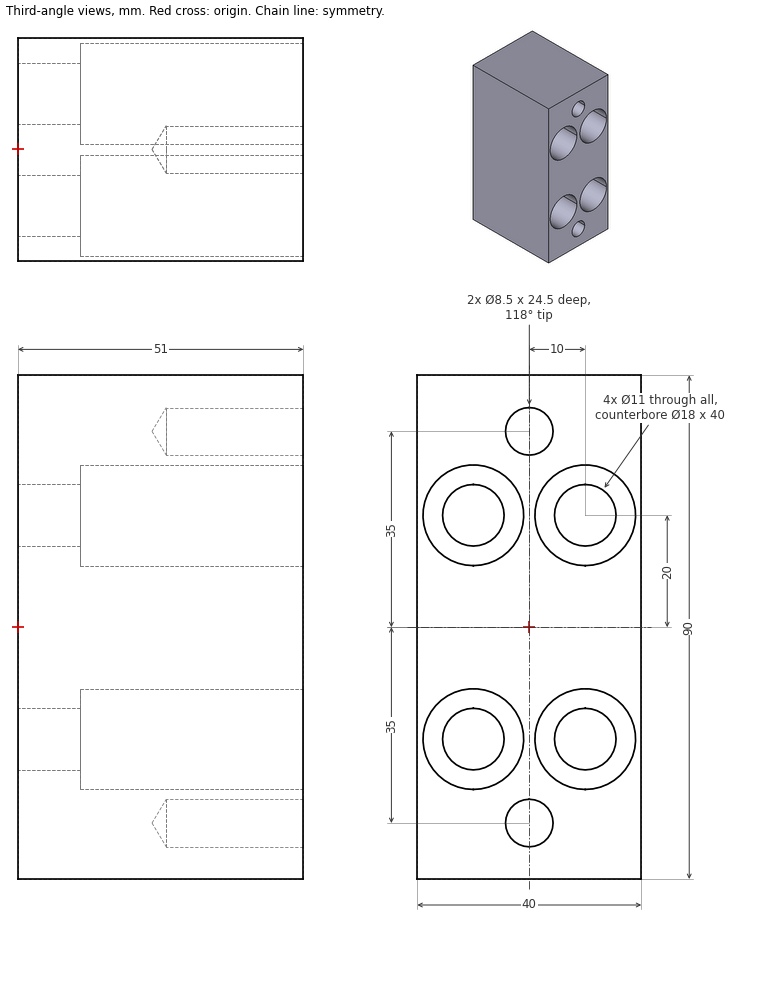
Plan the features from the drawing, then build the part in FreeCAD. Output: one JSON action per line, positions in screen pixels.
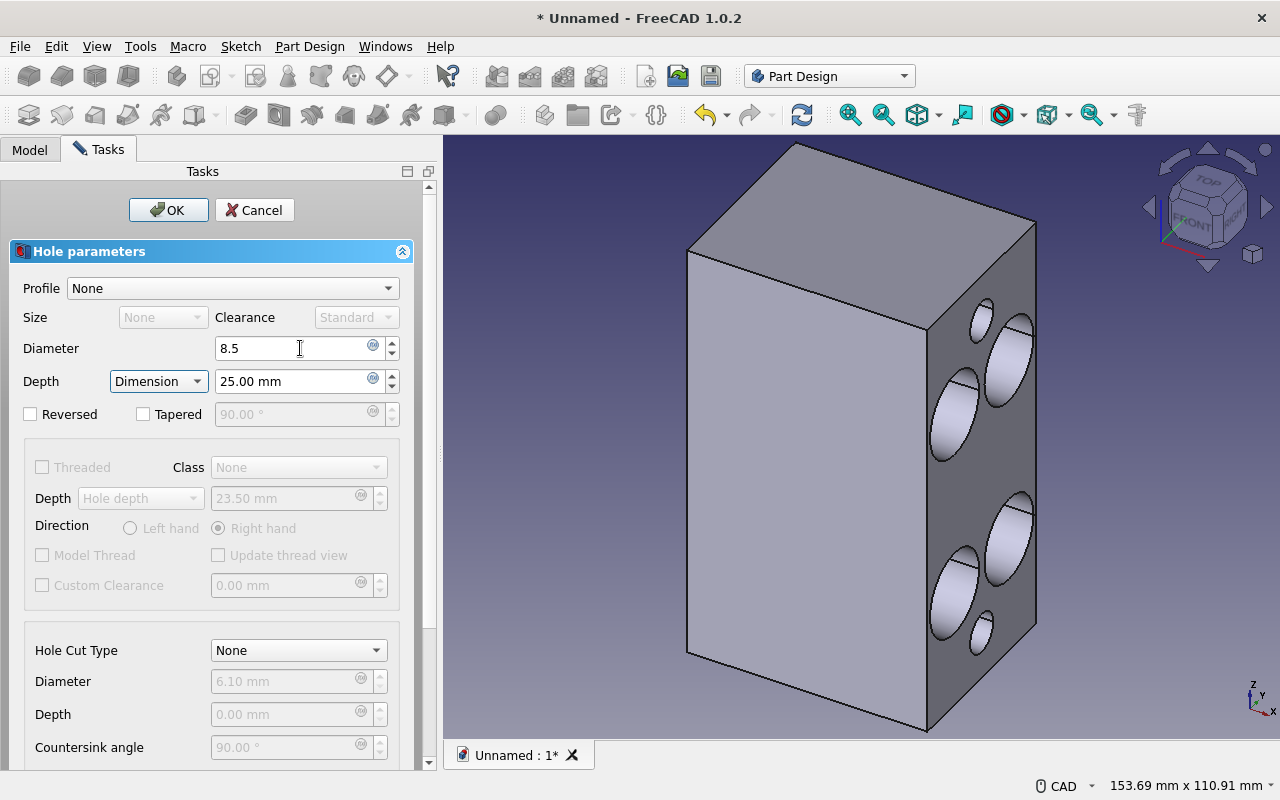
{"action": "triple_click", "coordinate": [300, 382]}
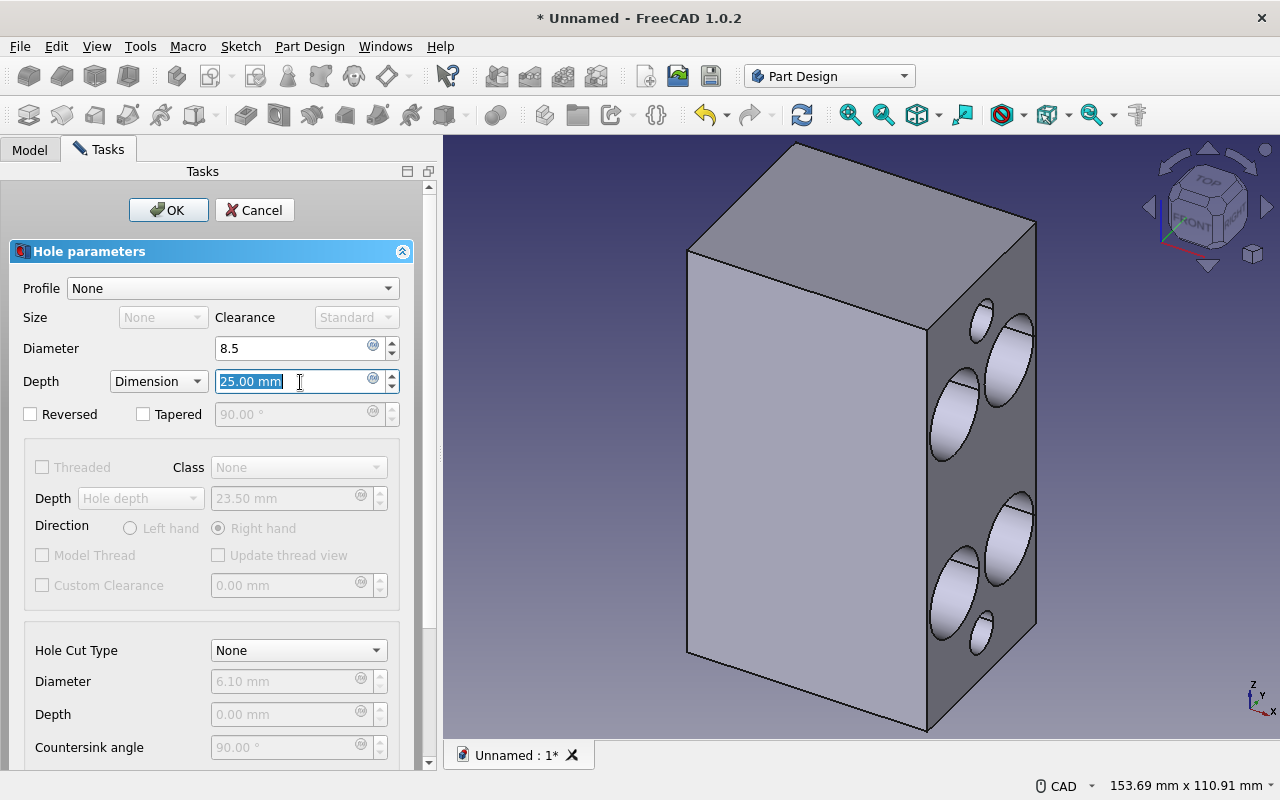
{"action": "type", "text": "24.5"}
{"action": "key", "text": "Tab"}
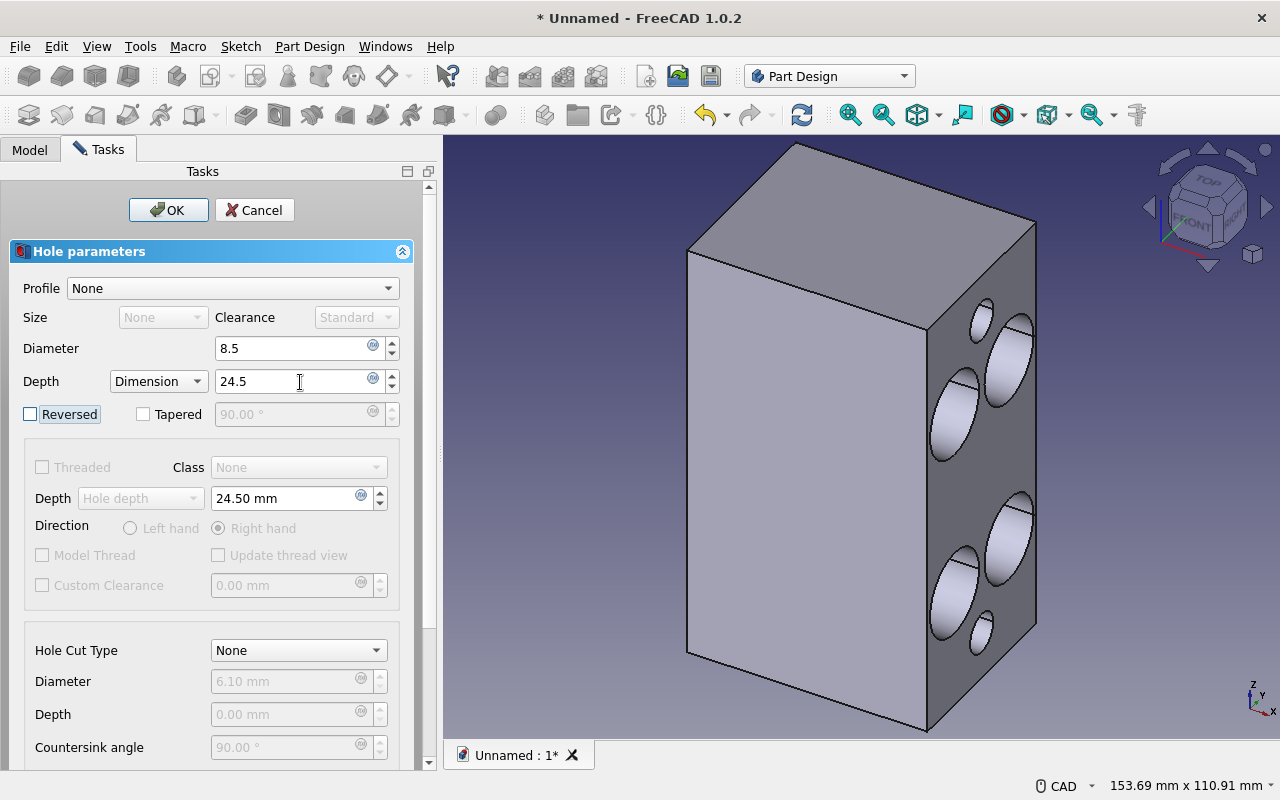
{"action": "left_click", "coordinate": [169, 210]}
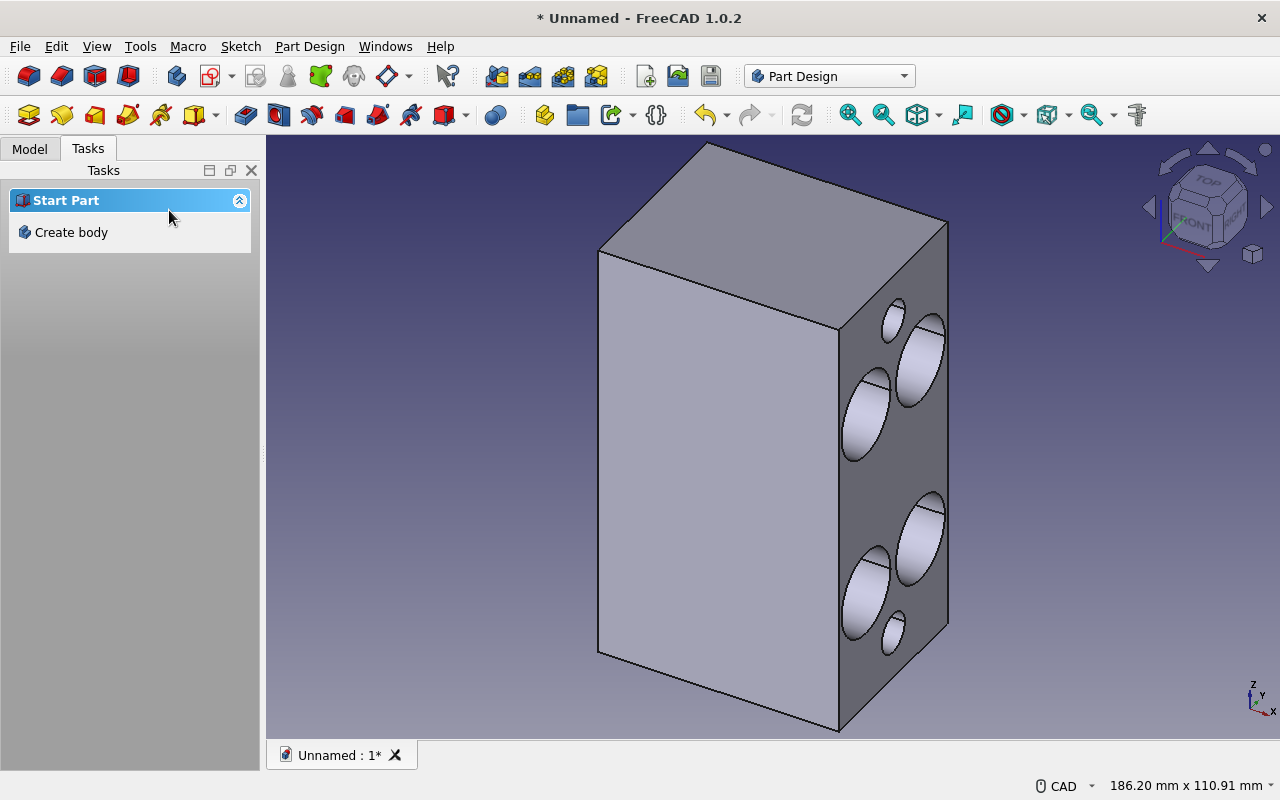
{"action": "key", "text": "0"}